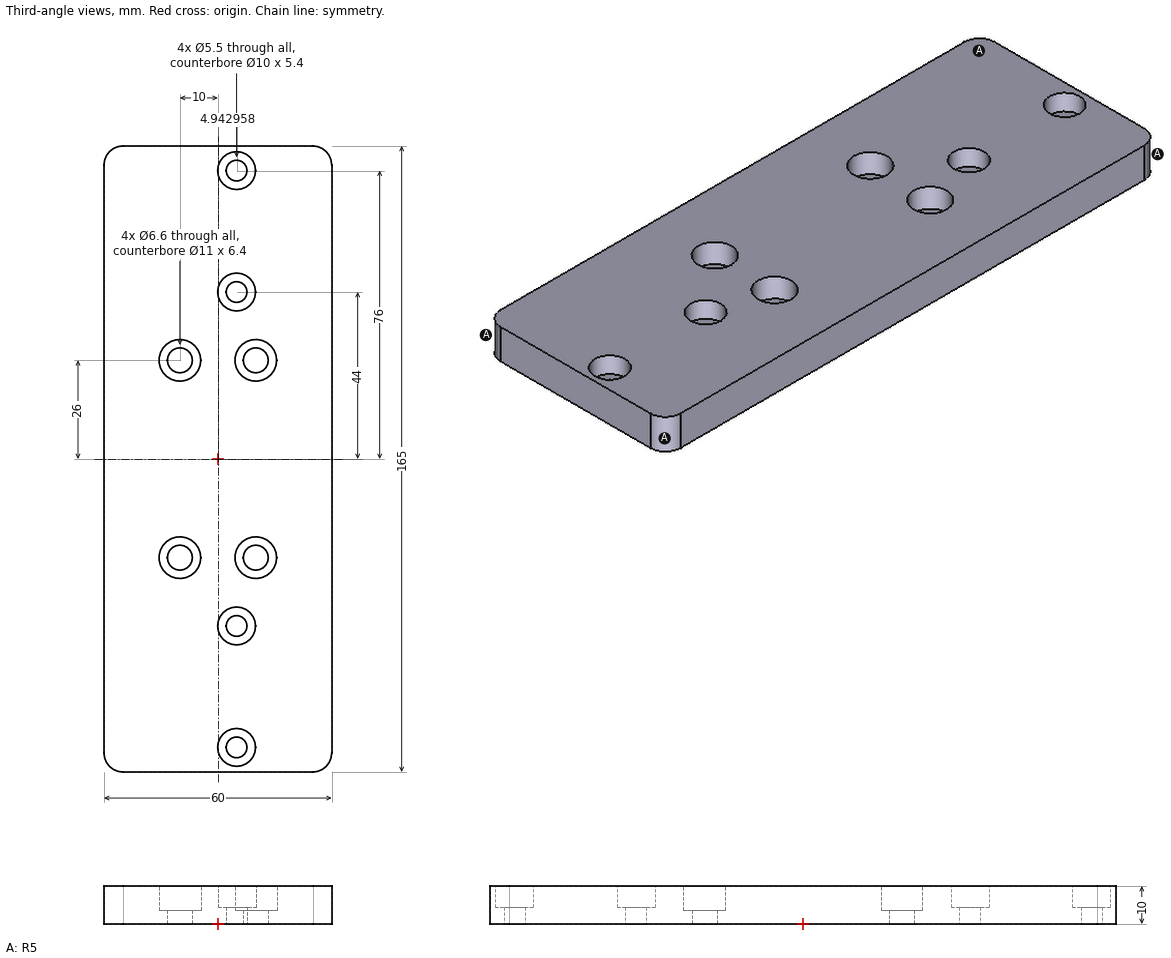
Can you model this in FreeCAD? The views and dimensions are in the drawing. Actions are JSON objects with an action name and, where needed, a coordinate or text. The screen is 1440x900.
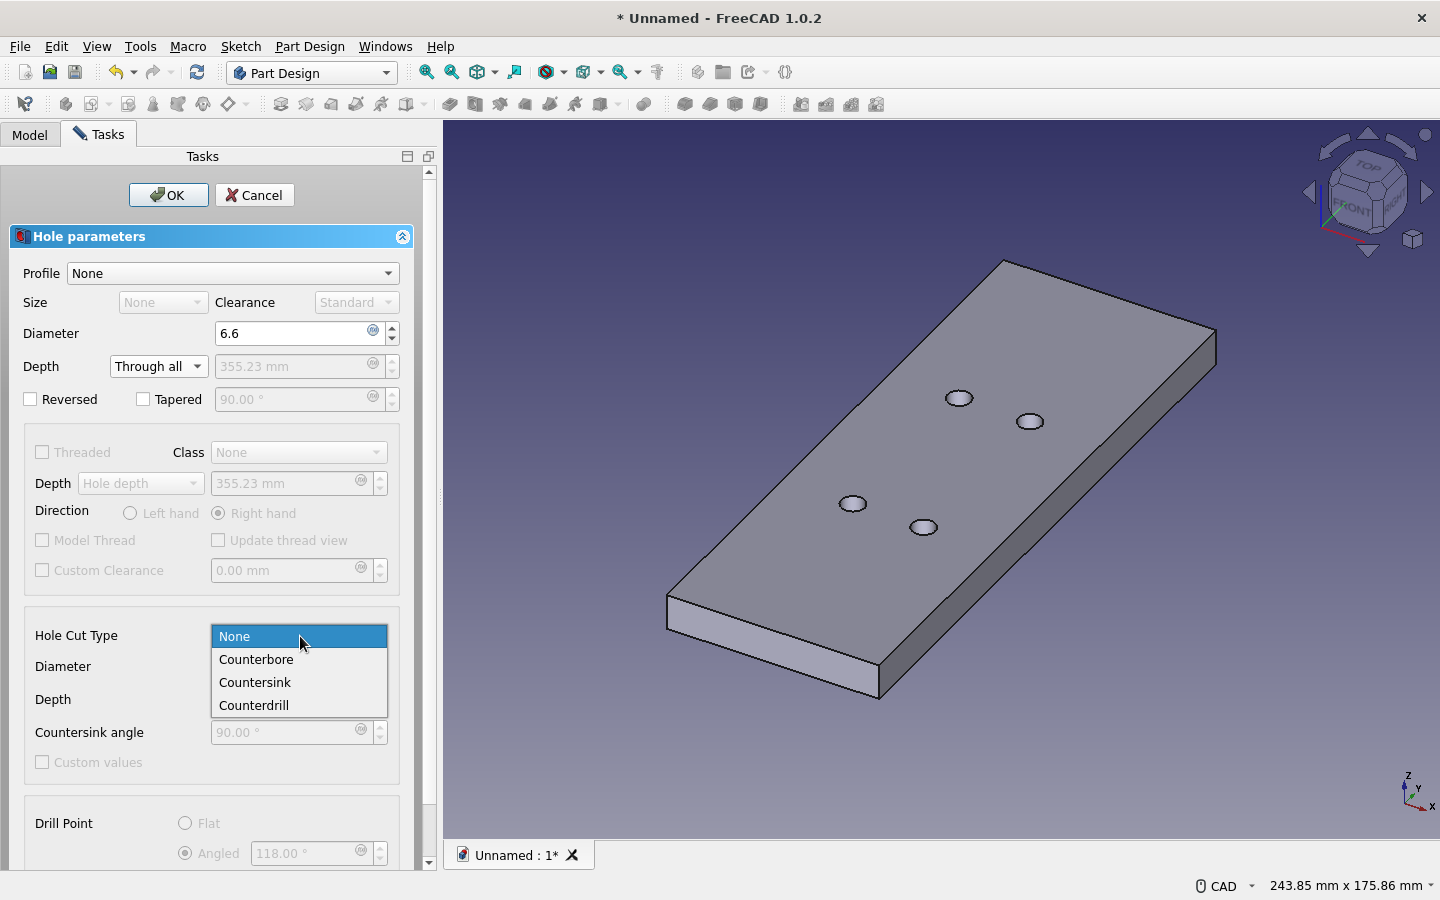
{"action": "left_click", "coordinate": [298, 660]}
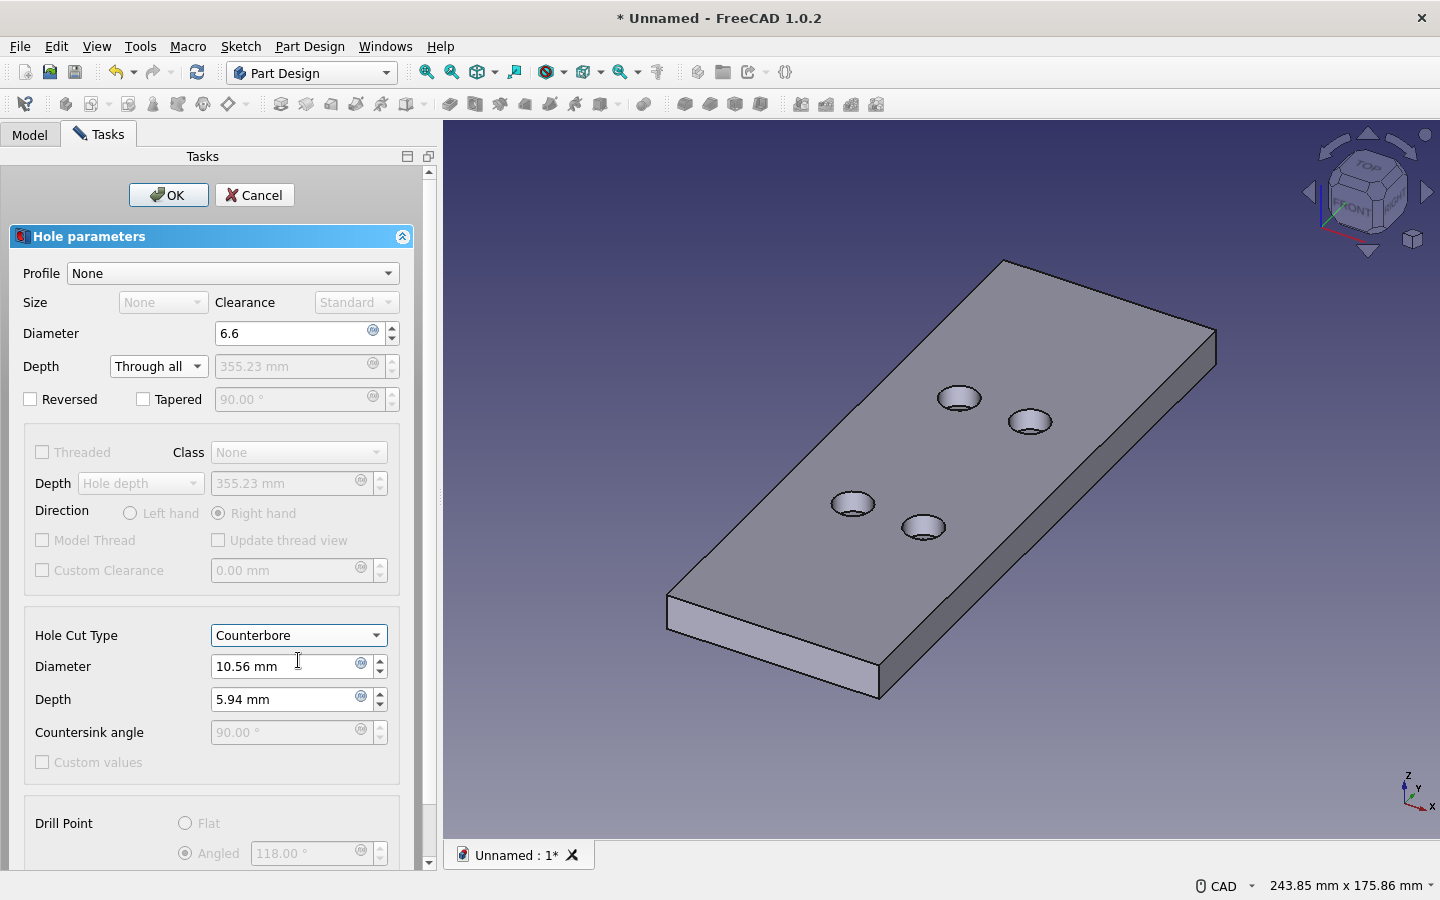
{"action": "triple_click", "coordinate": [292, 666]}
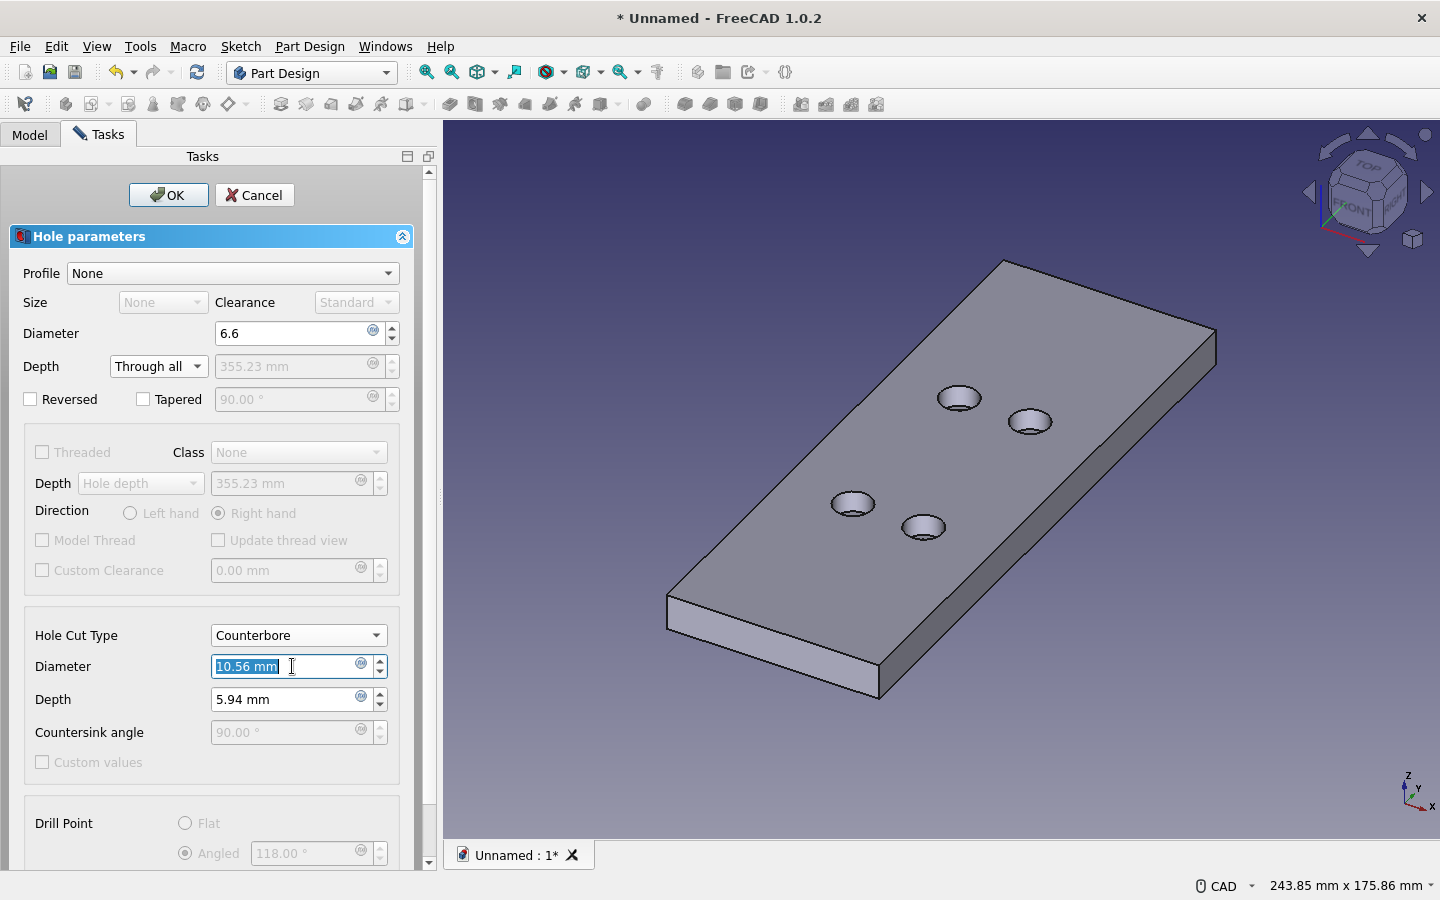
{"action": "type", "text": "11"}
{"action": "key", "text": "Tab"}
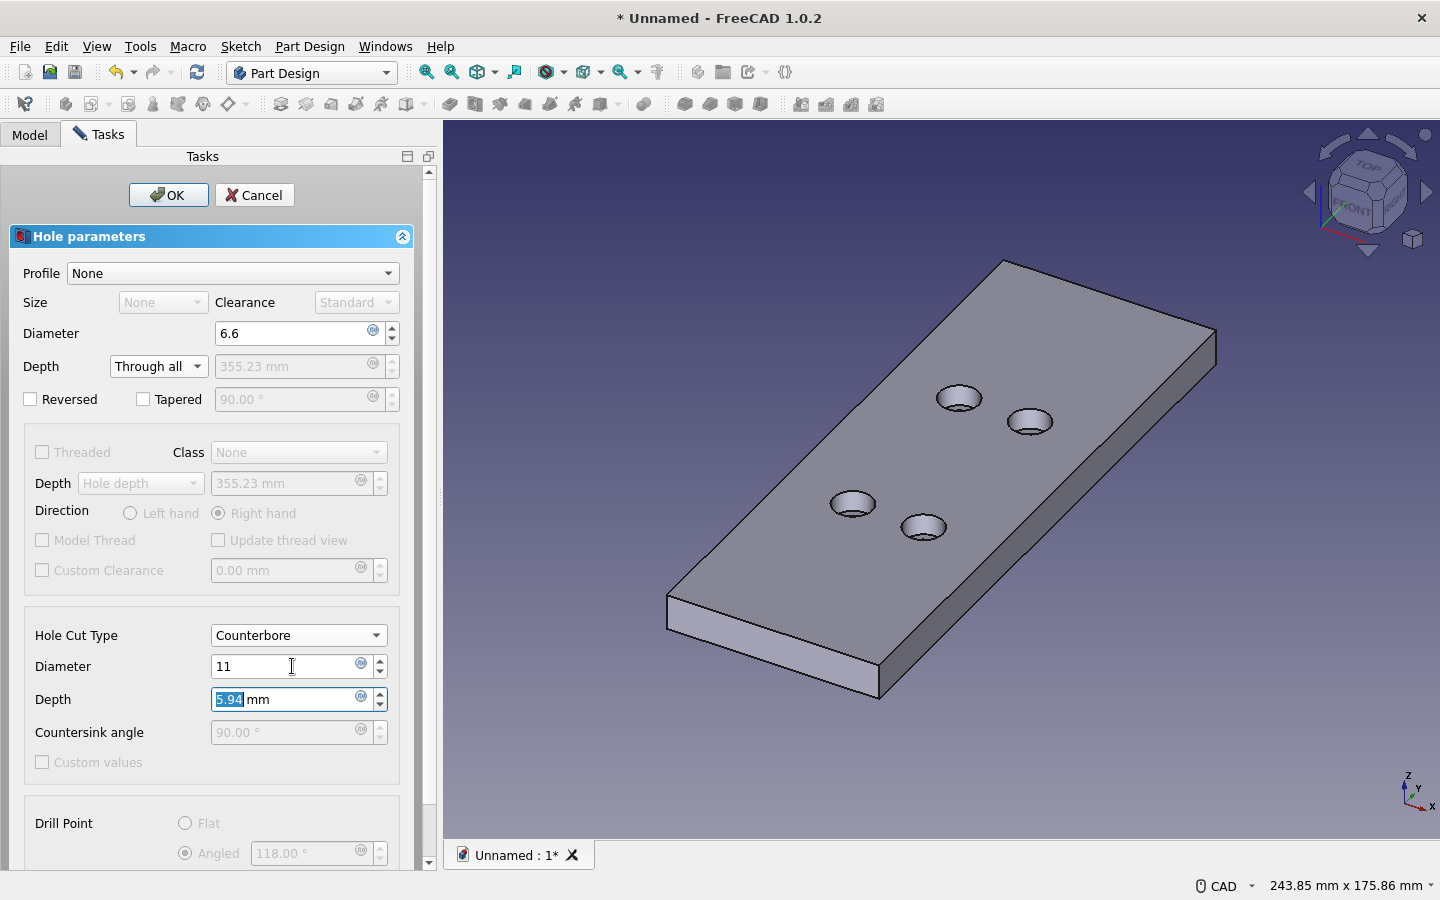
{"action": "type", "text": "6.4"}
{"action": "key", "text": "Tab"}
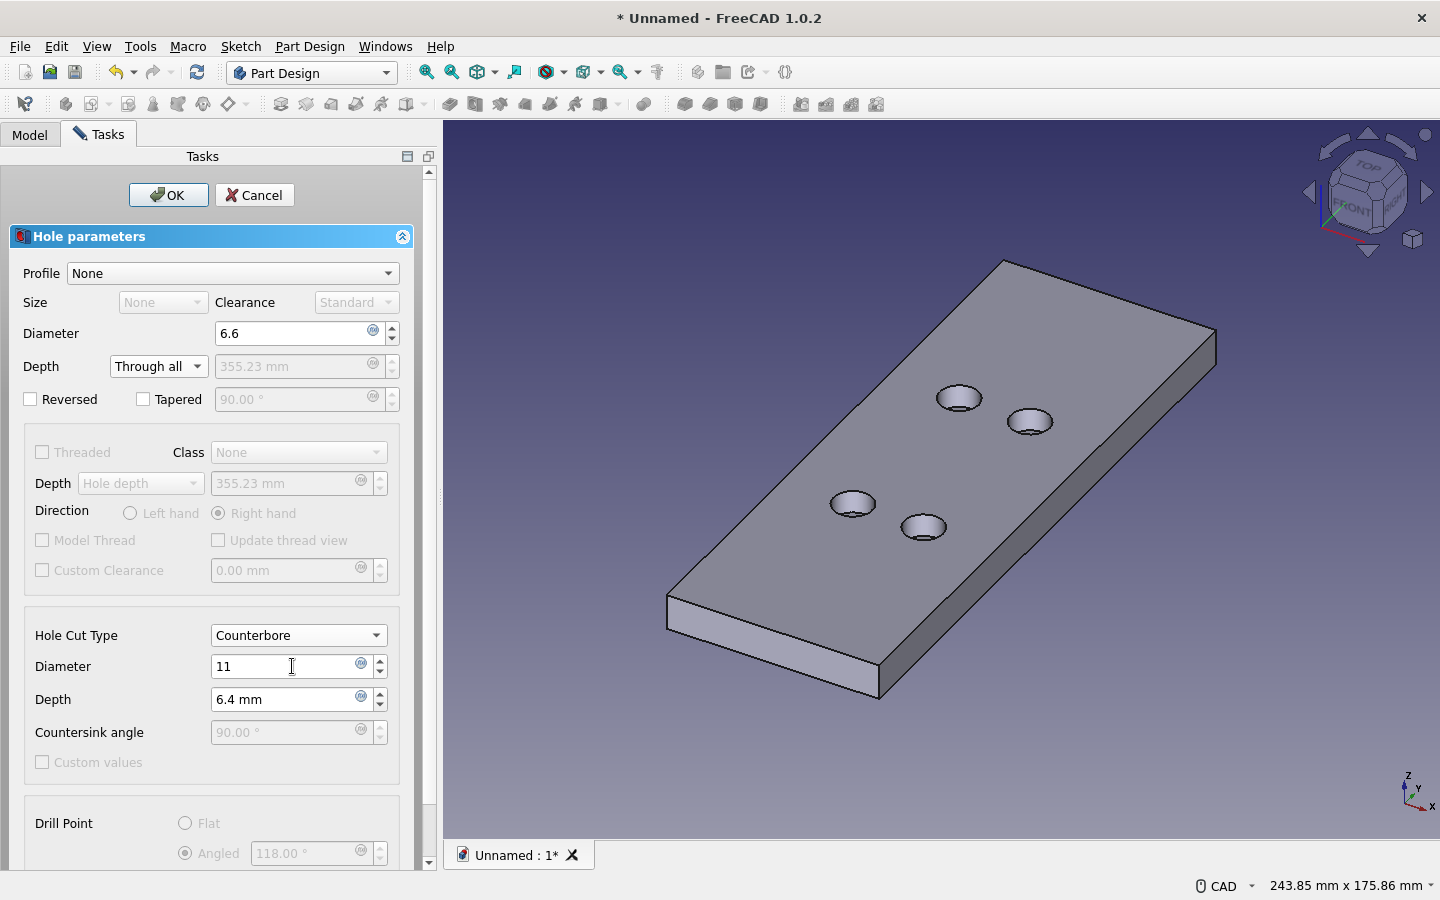
{"action": "left_click", "coordinate": [169, 195]}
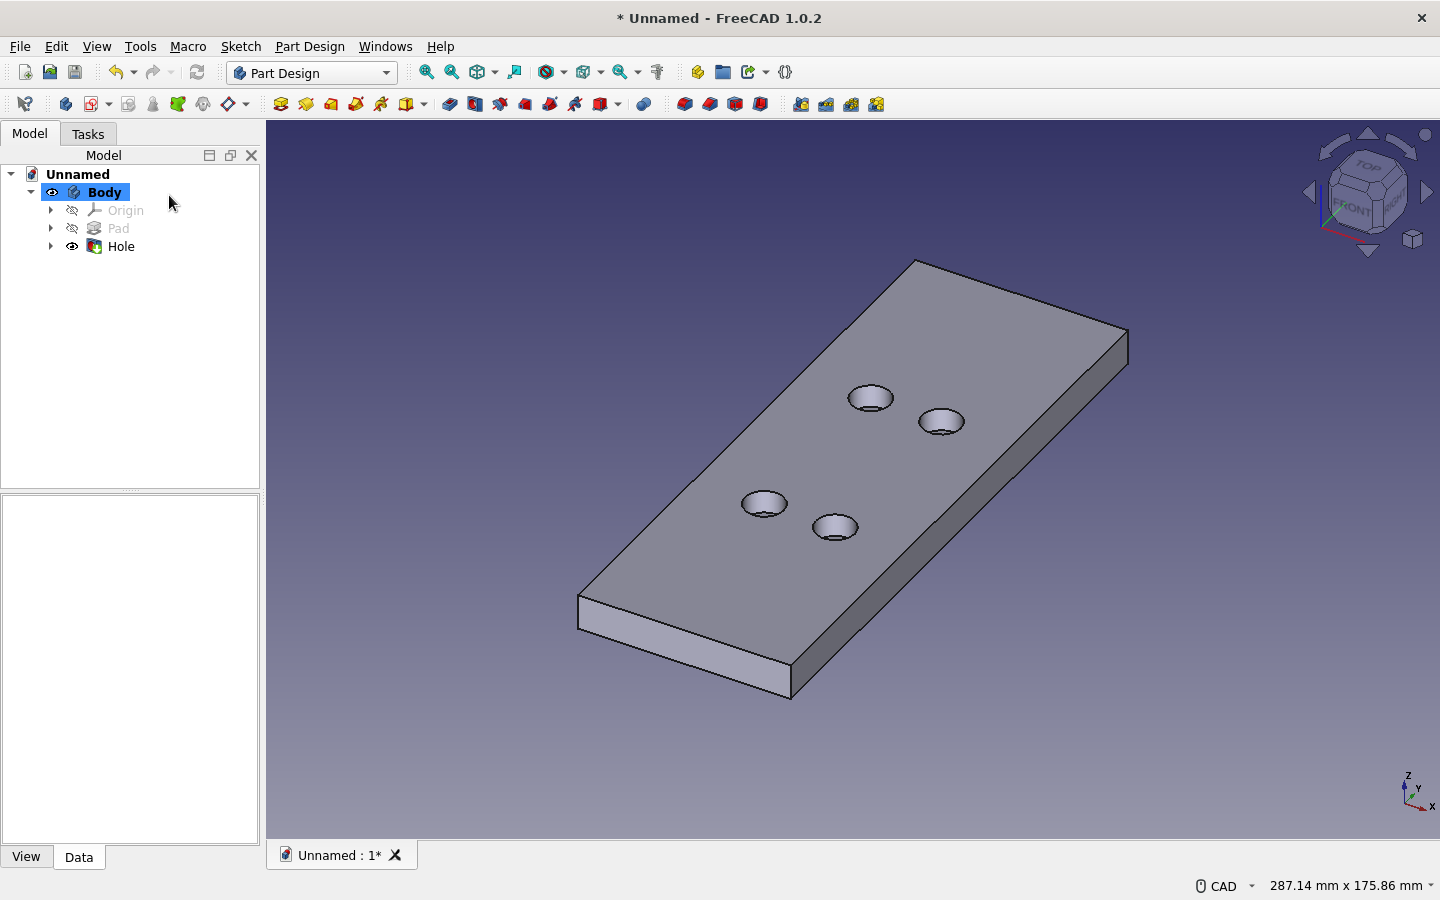
{"action": "left_click", "coordinate": [853, 462]}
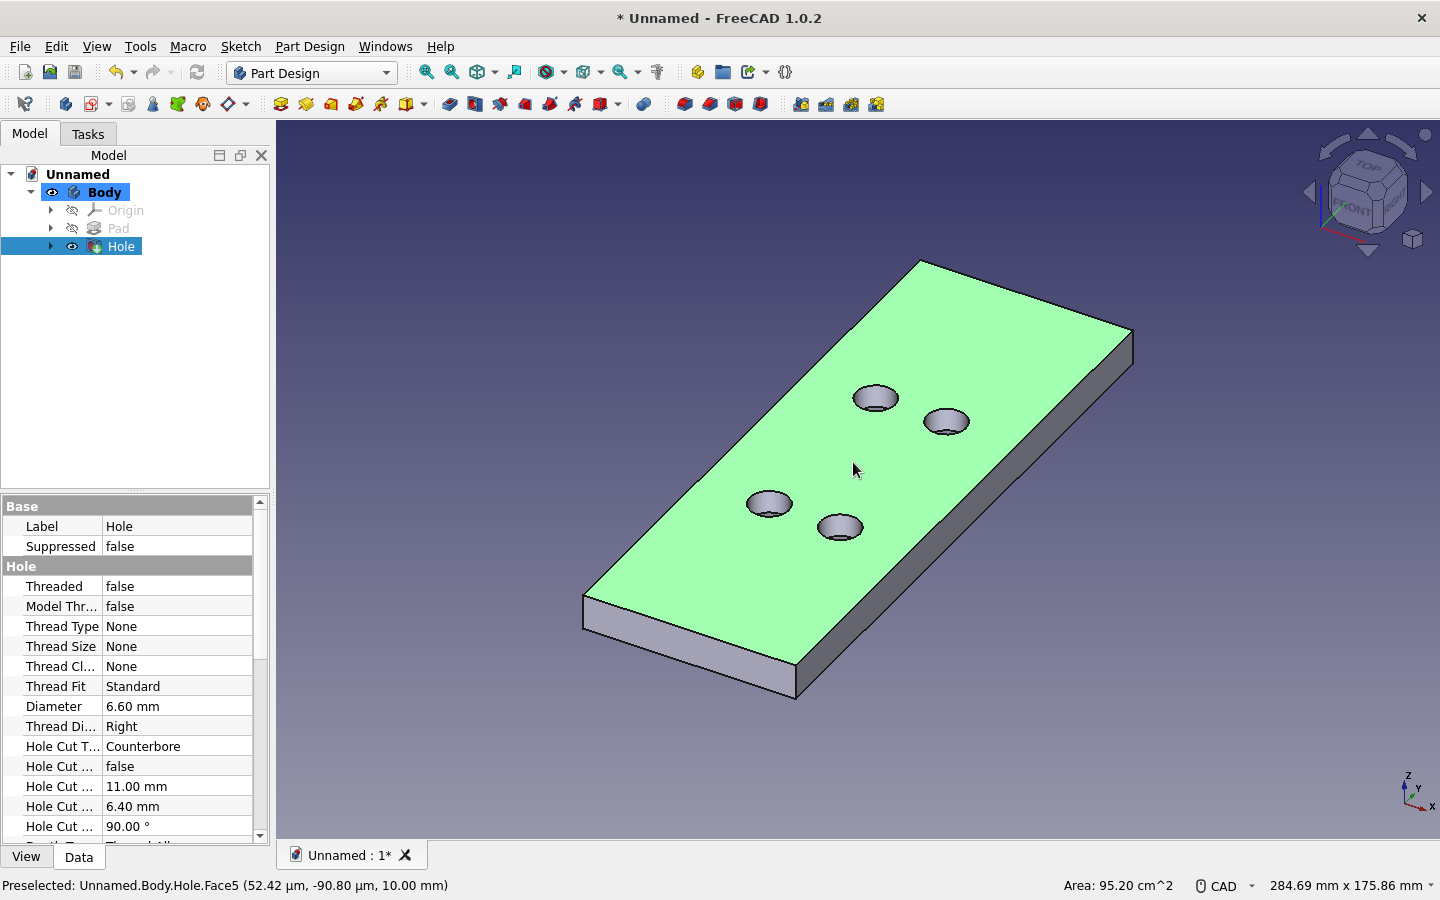
{"action": "left_click", "coordinate": [90, 104]}